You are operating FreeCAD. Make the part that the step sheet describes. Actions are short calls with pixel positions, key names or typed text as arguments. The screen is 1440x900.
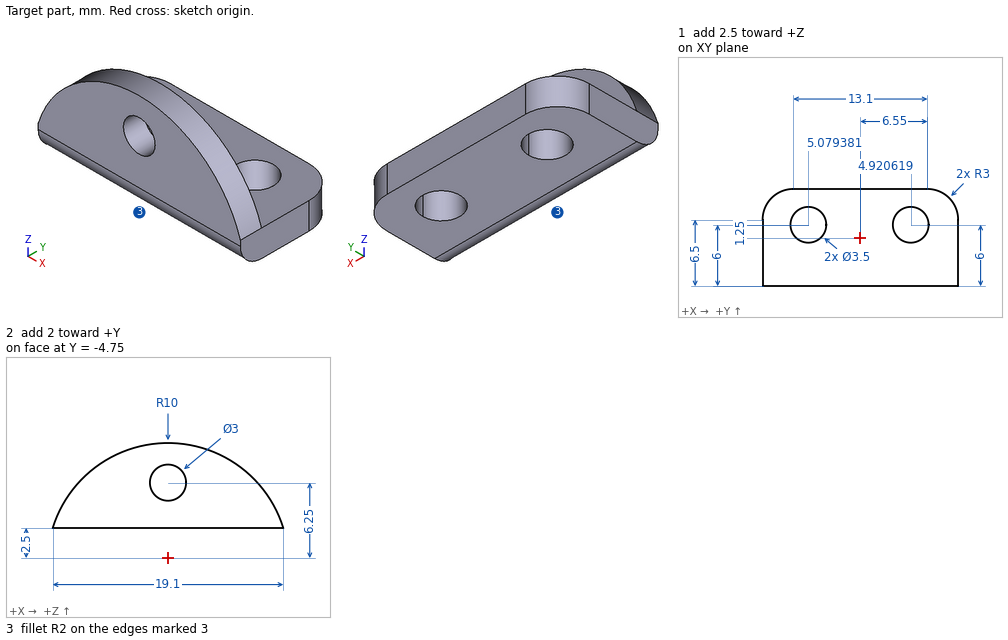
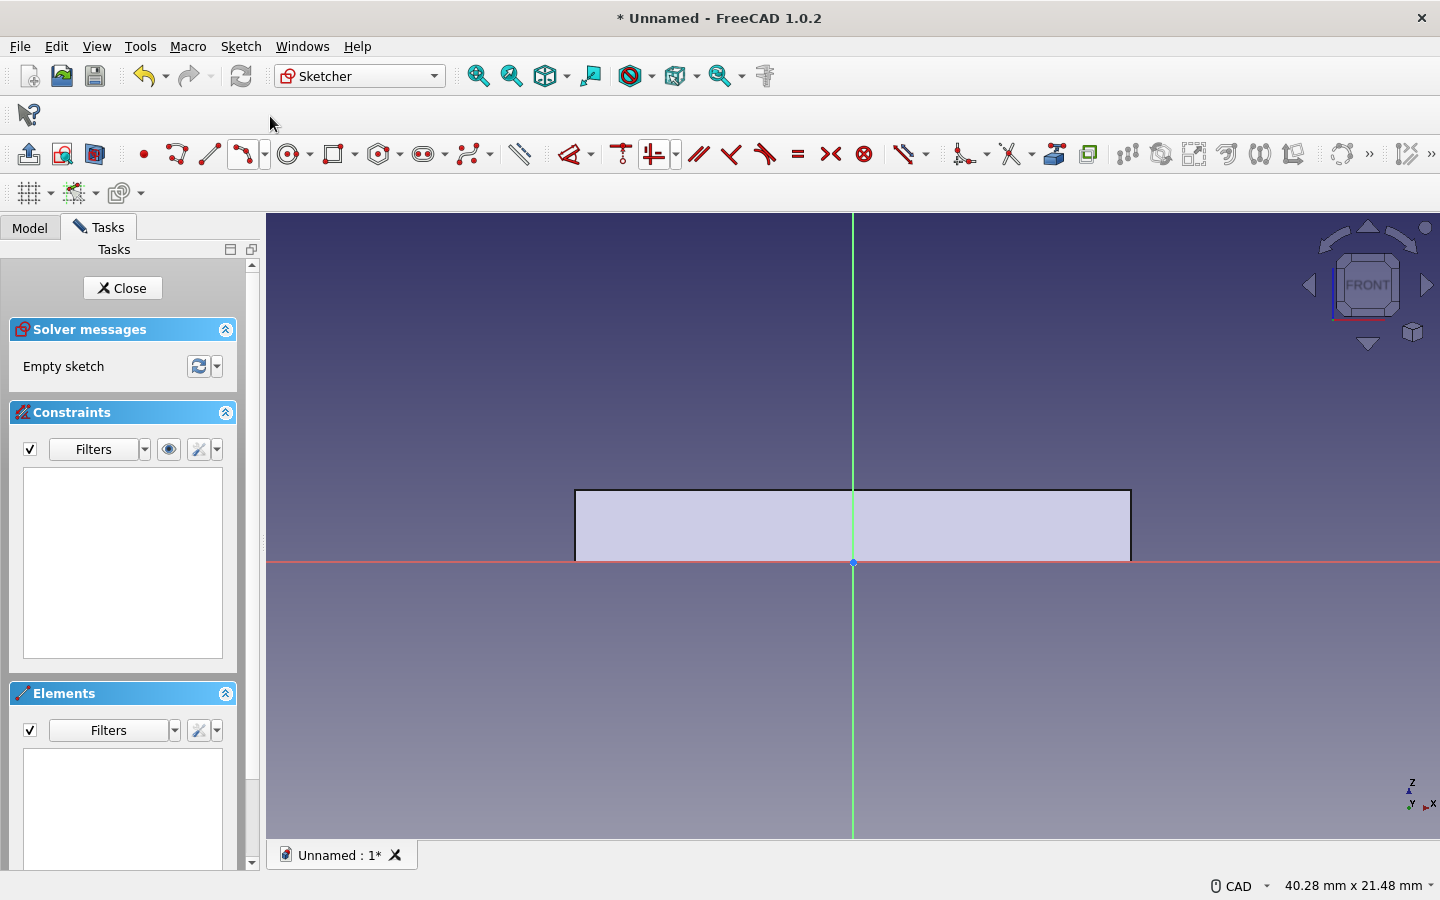
click(210, 154)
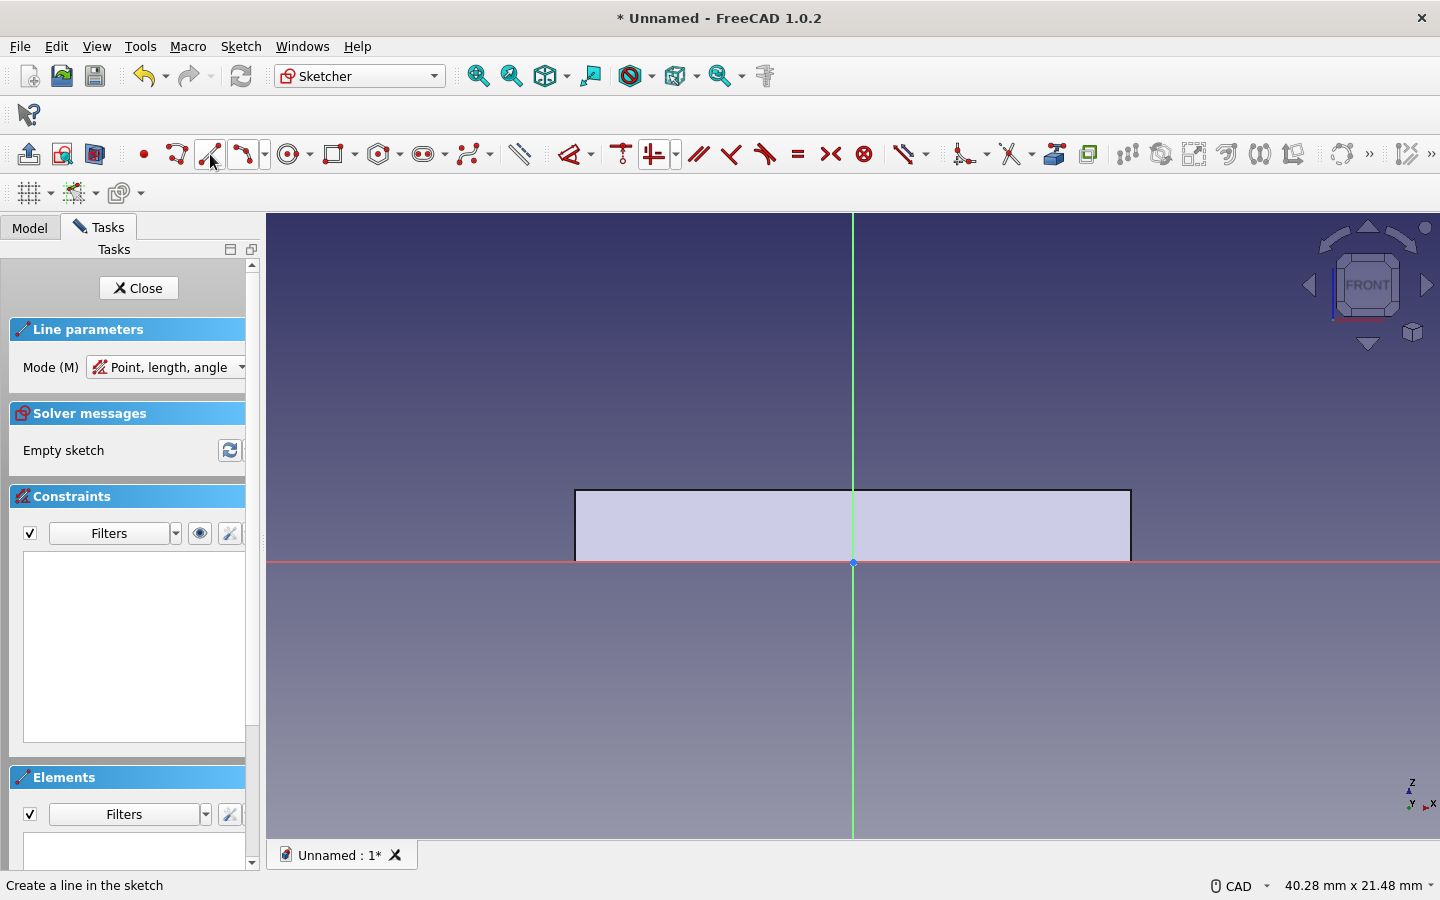
click(575, 490)
click(1131, 490)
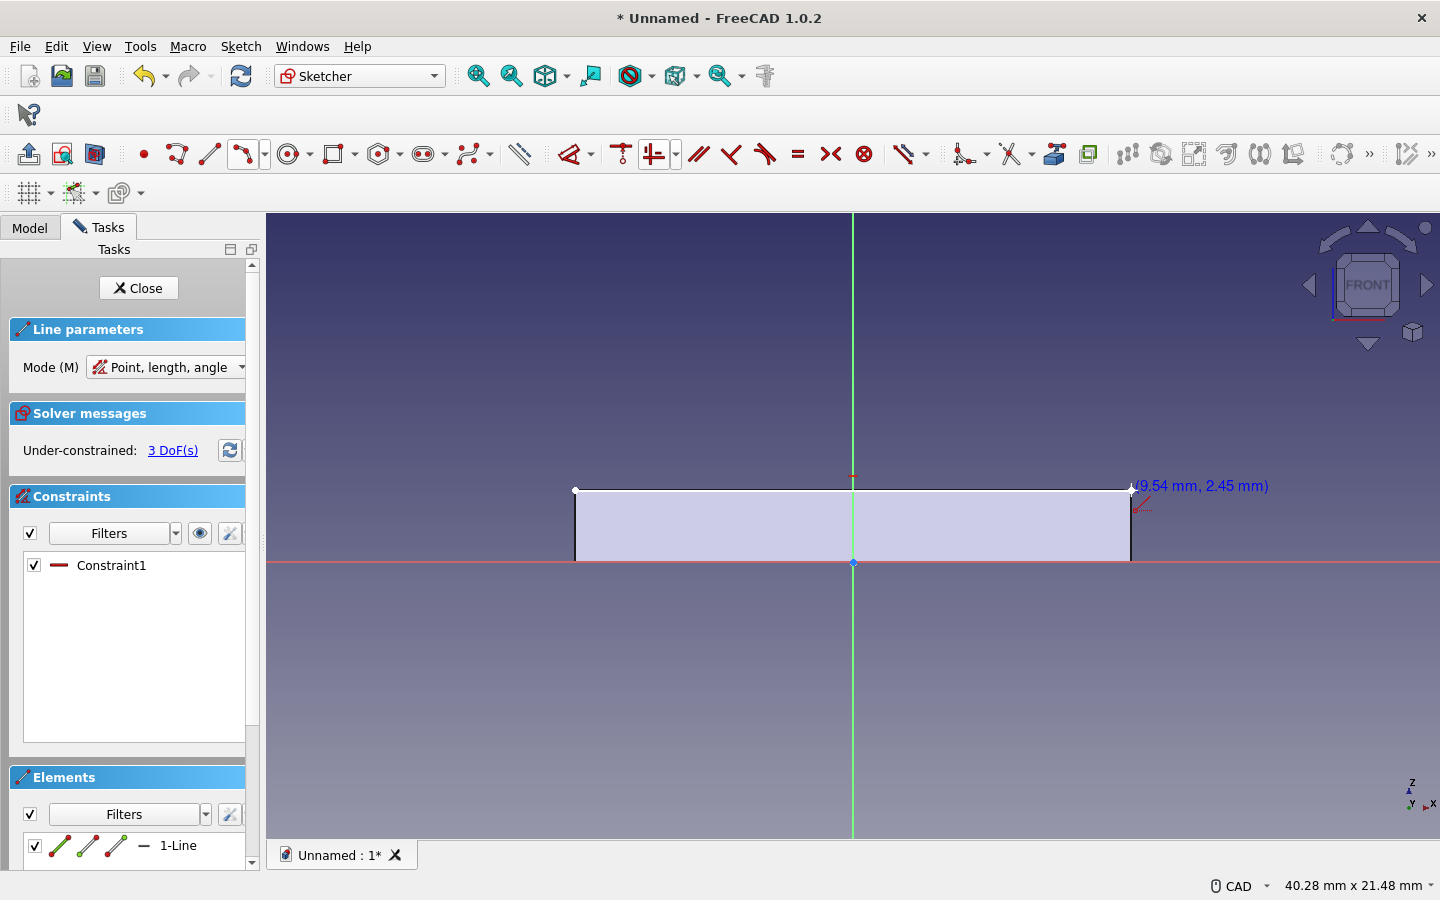
click(242, 154)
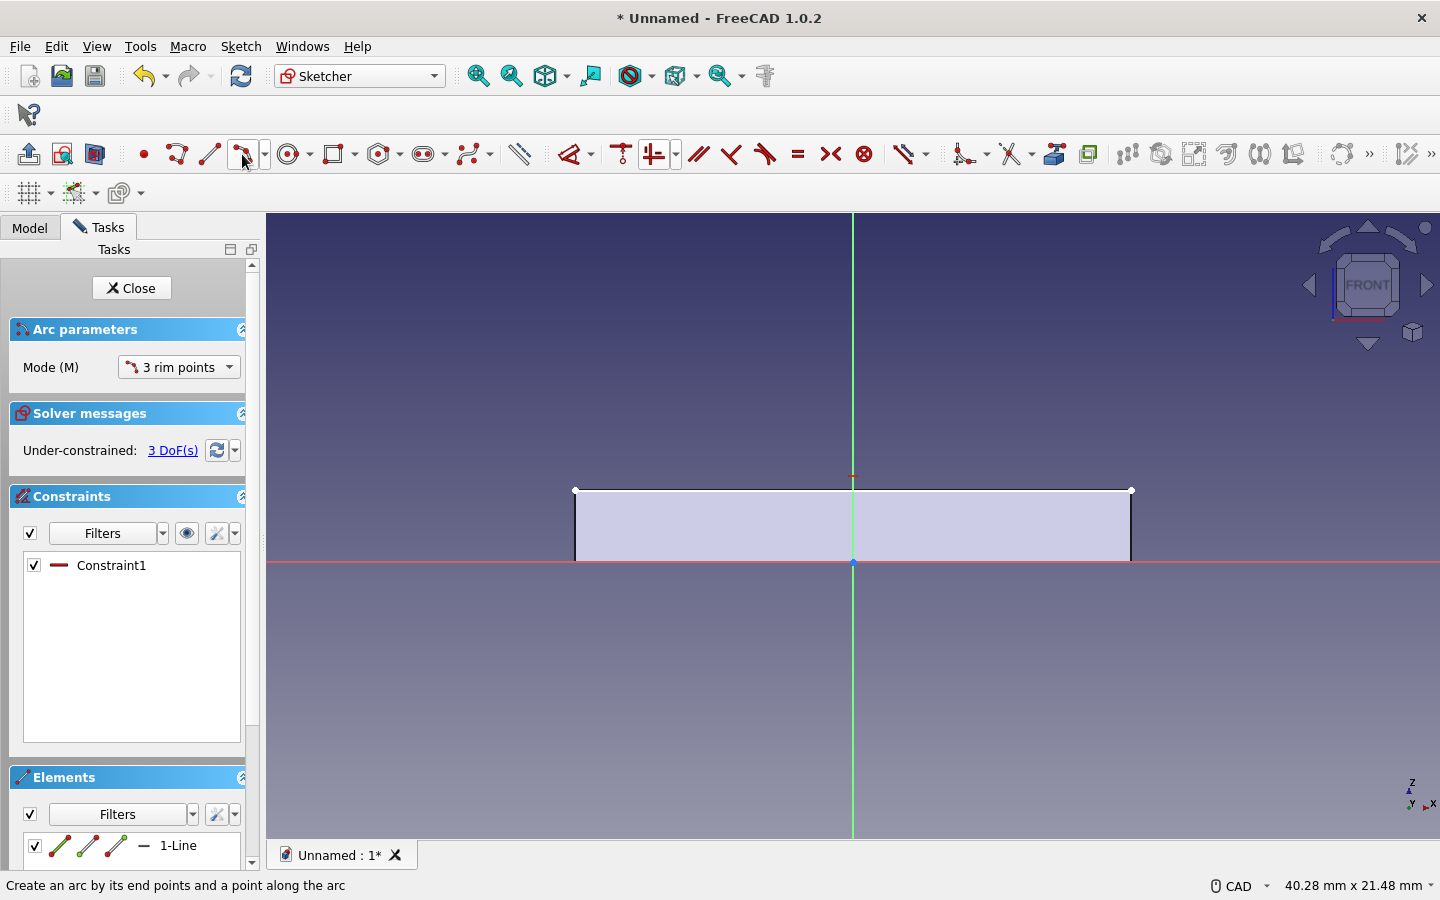
click(1131, 491)
click(575, 491)
click(926, 294)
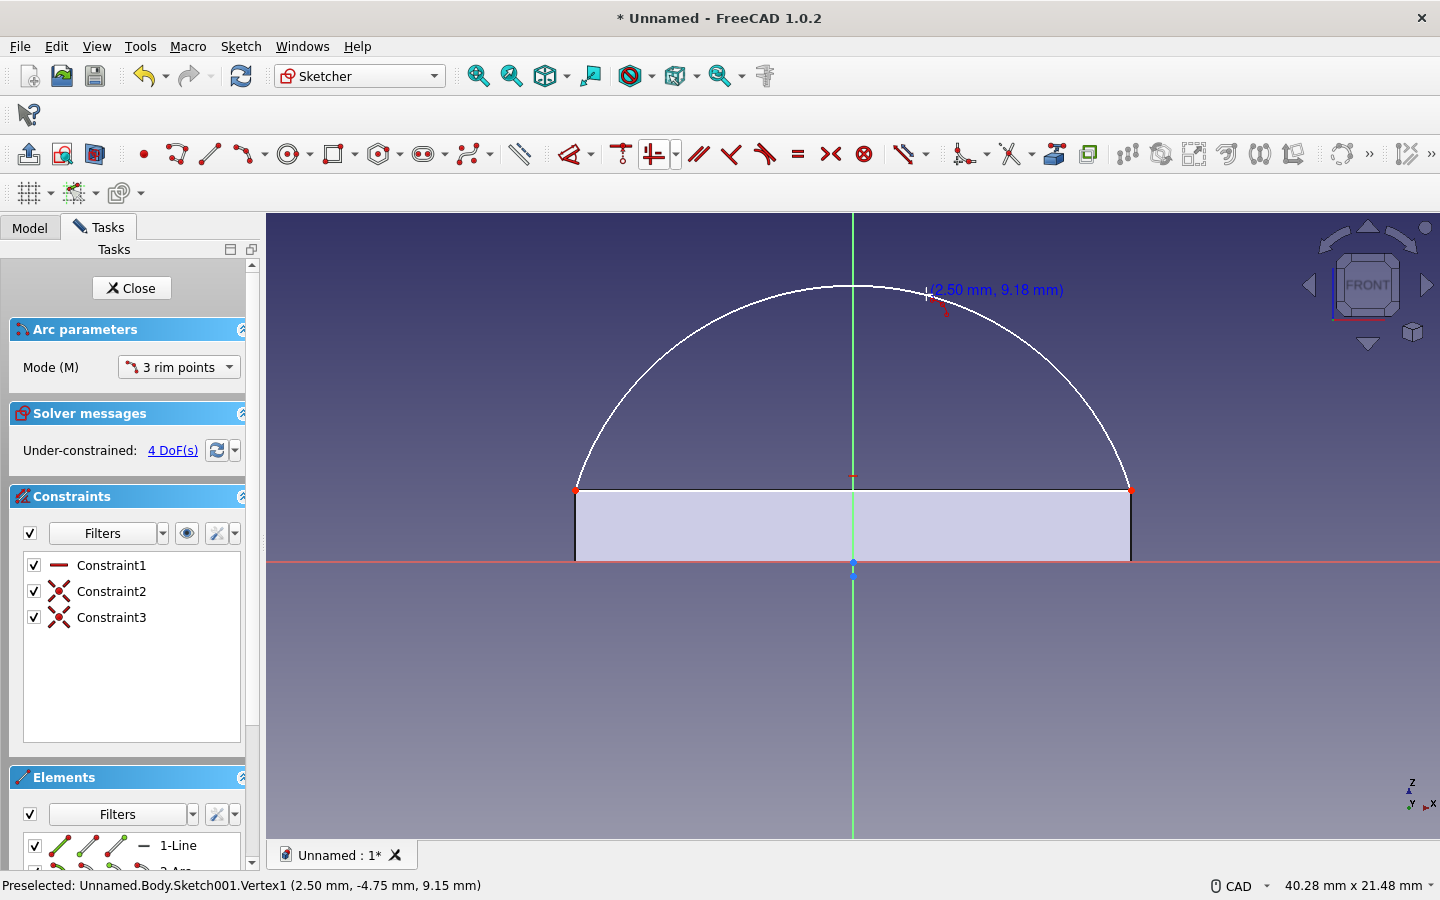
click(288, 154)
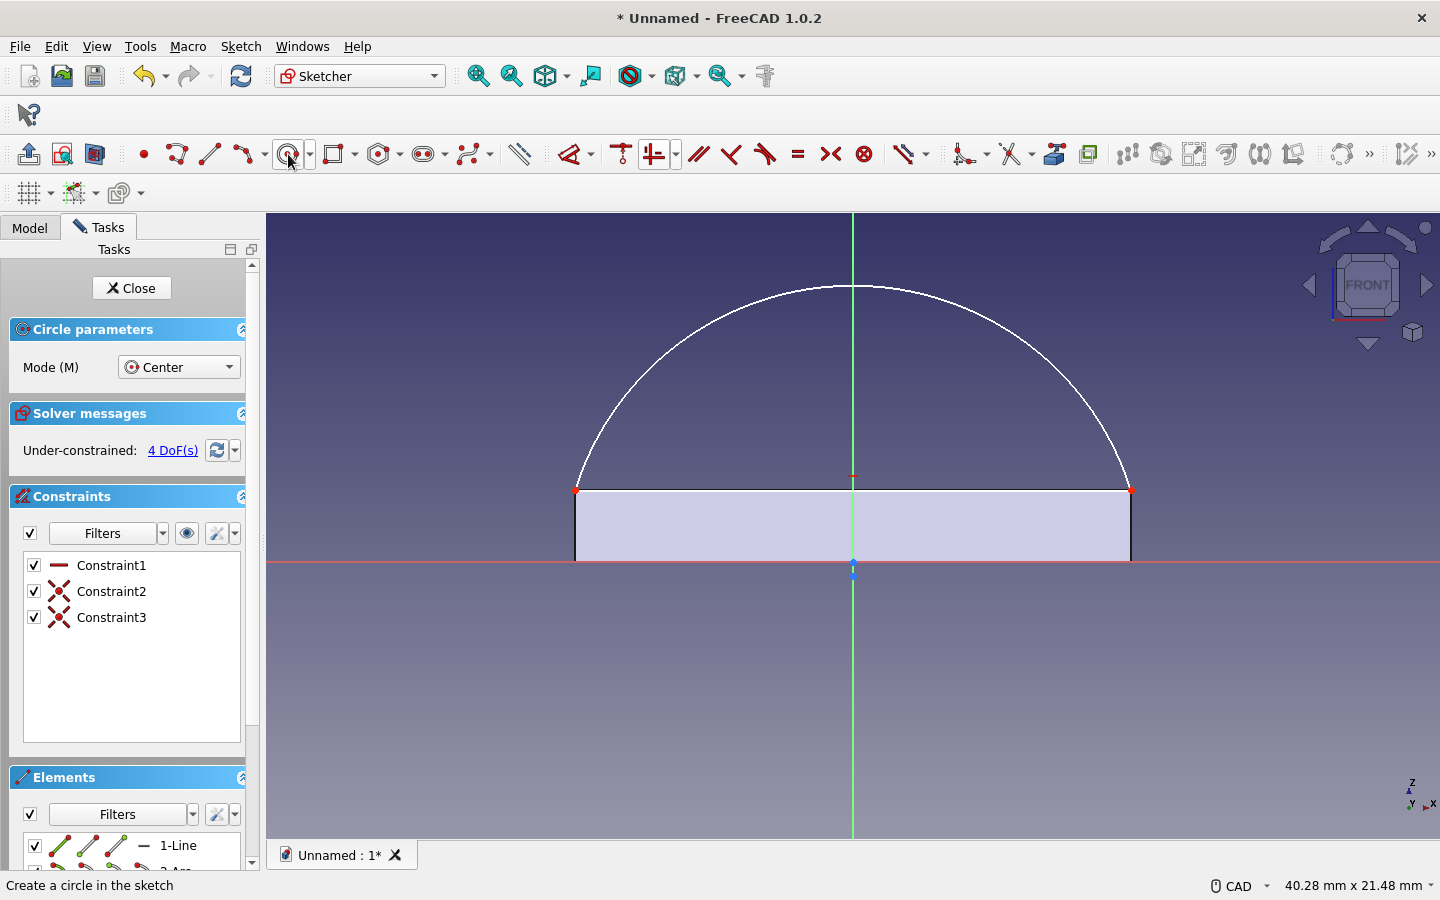
click(853, 380)
click(884, 349)
key(Escape)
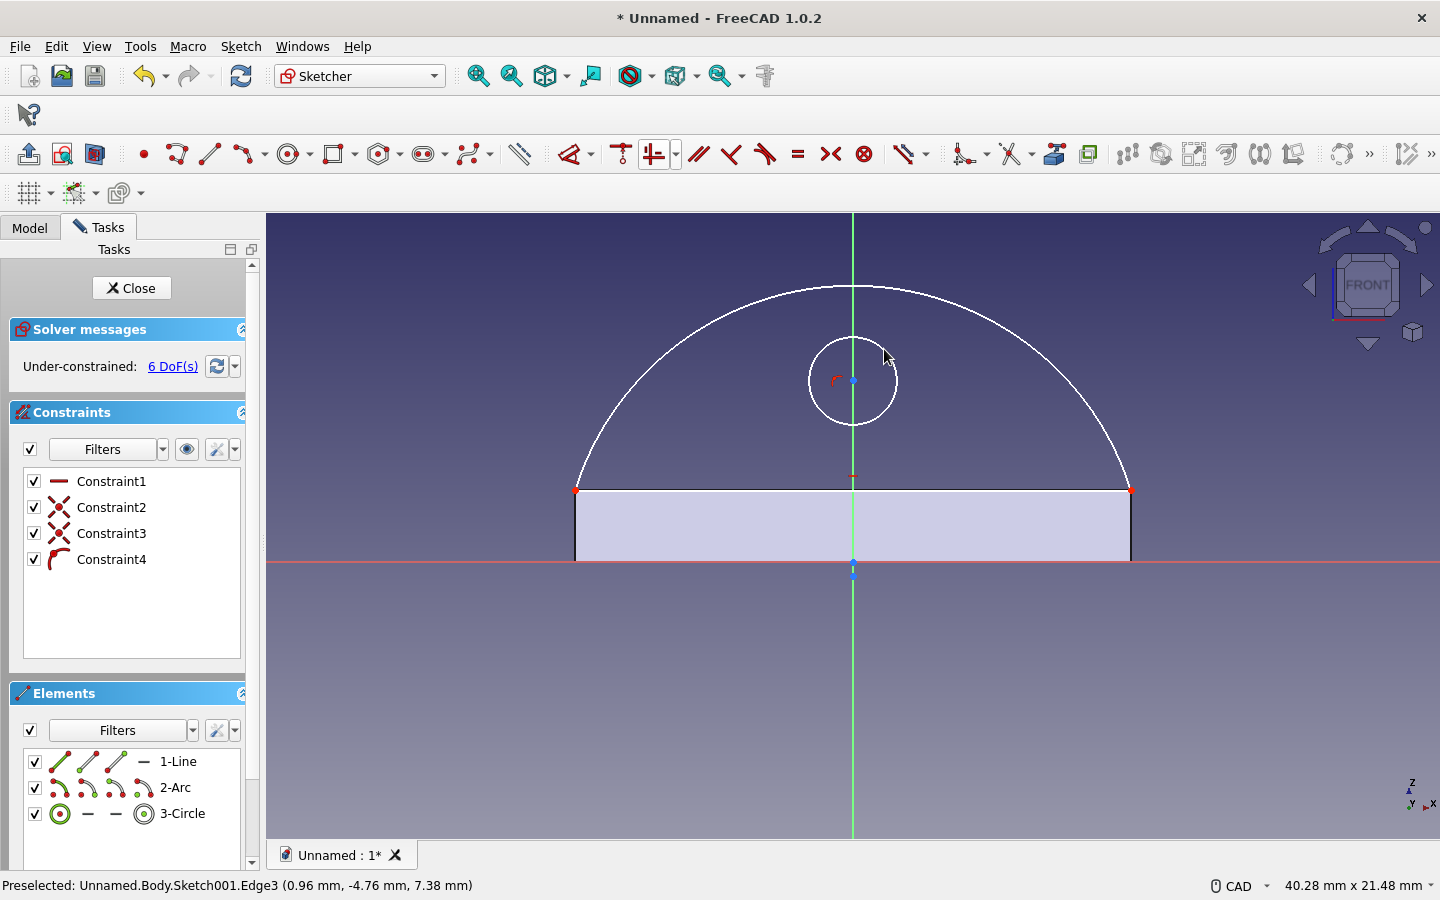
click(853, 577)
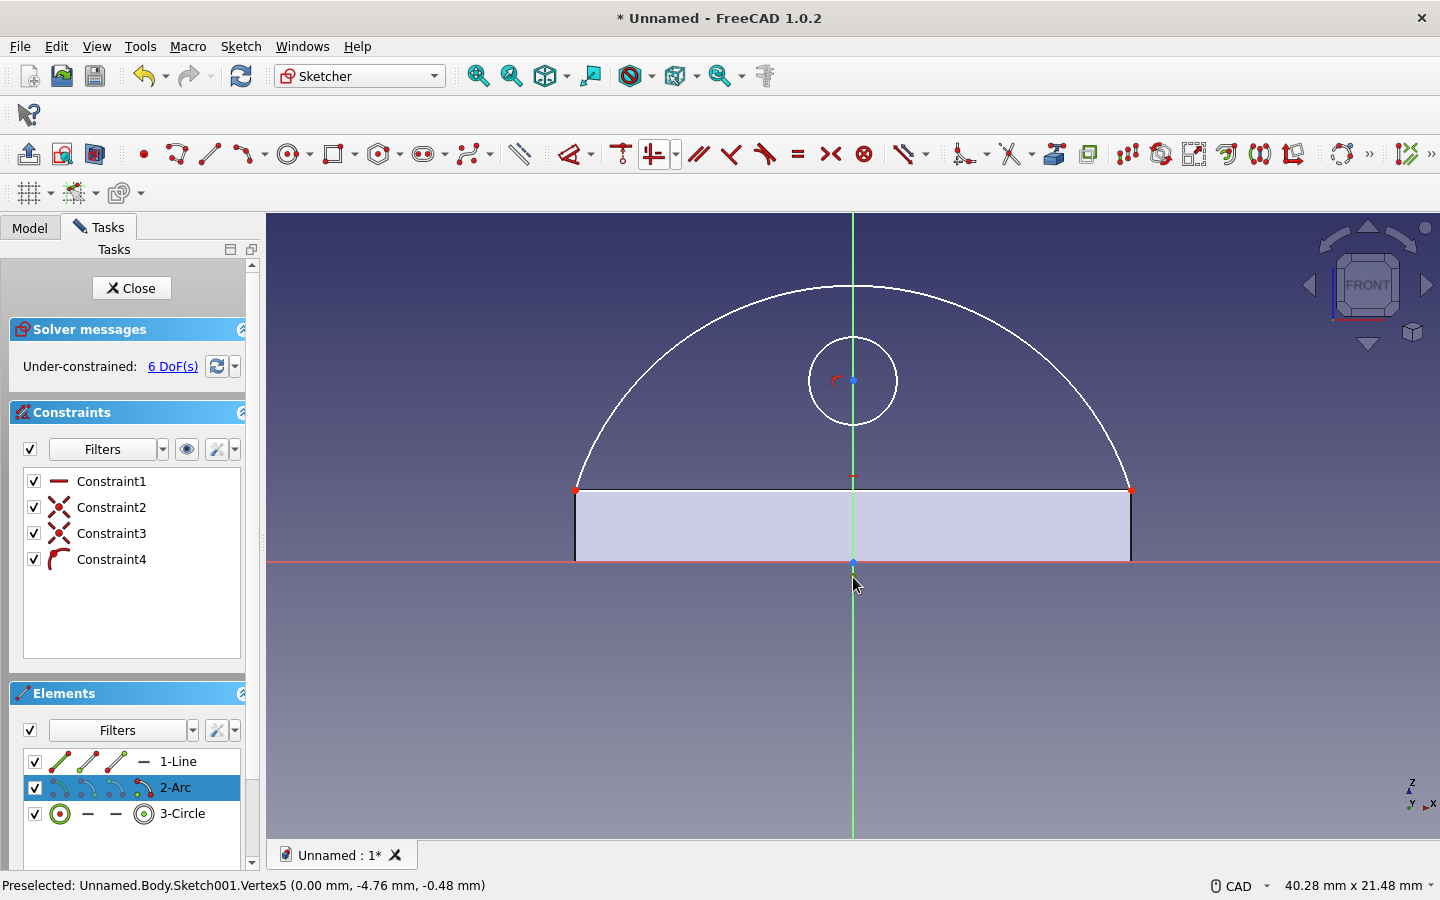
click(853, 770)